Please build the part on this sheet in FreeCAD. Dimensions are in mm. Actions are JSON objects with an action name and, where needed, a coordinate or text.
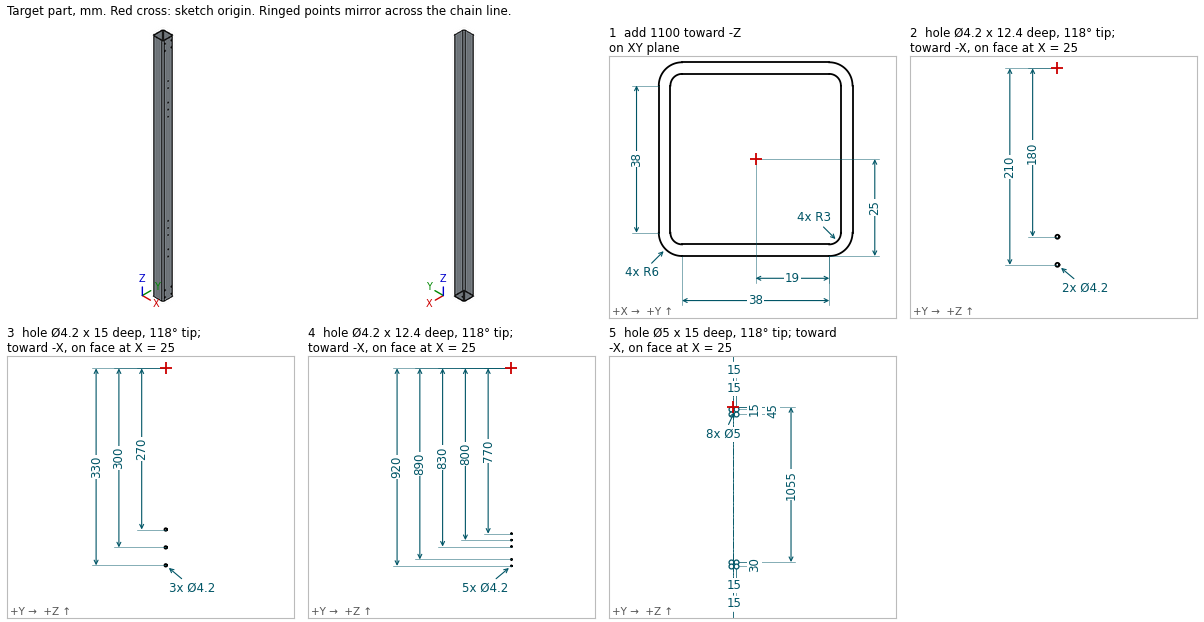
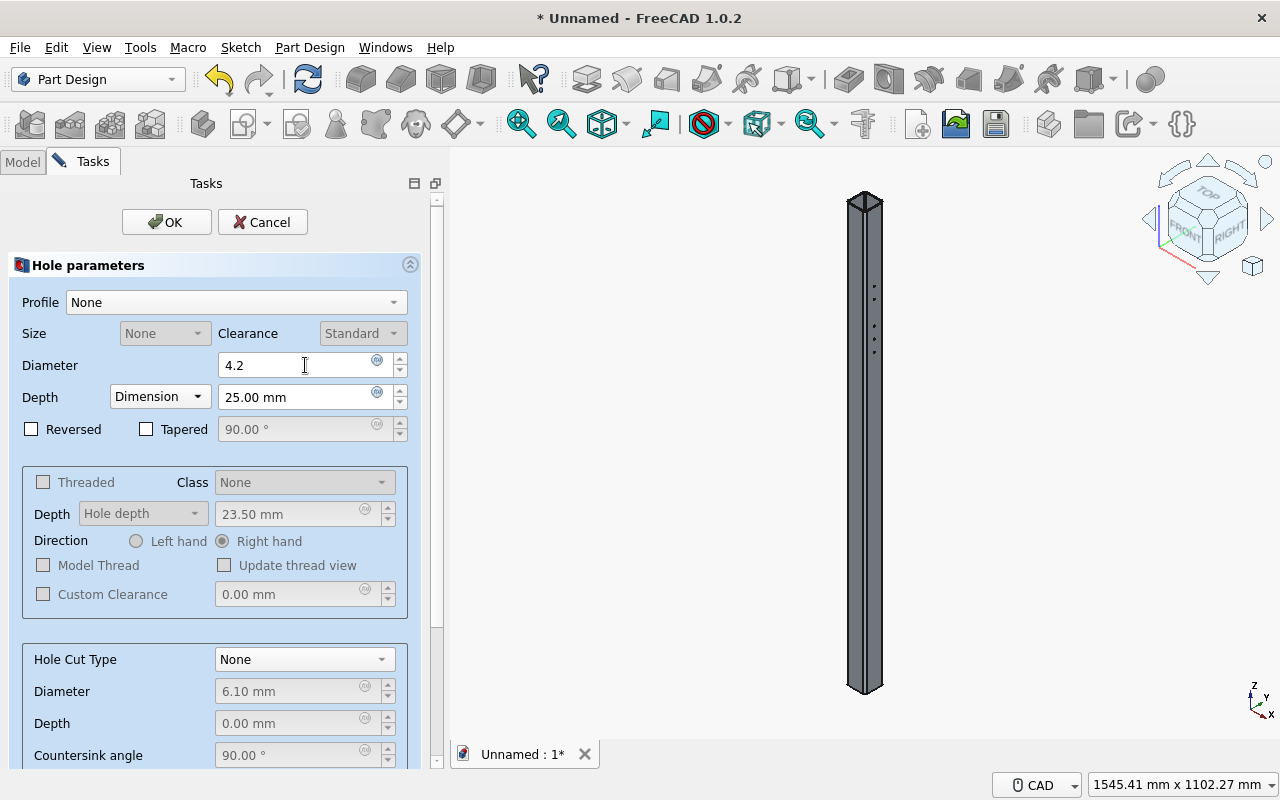
{"action": "triple_click", "coordinate": [305, 397]}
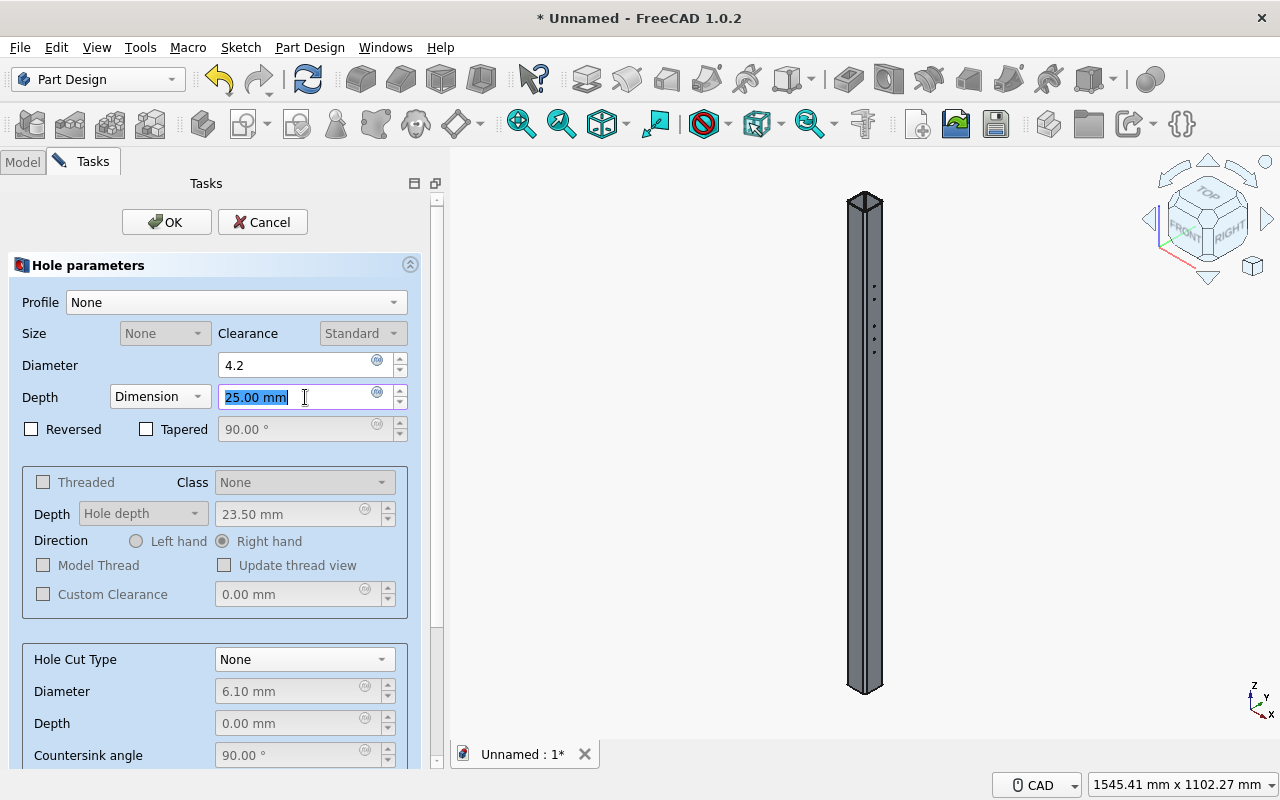
{"action": "type", "text": "15"}
{"action": "key", "text": "Tab"}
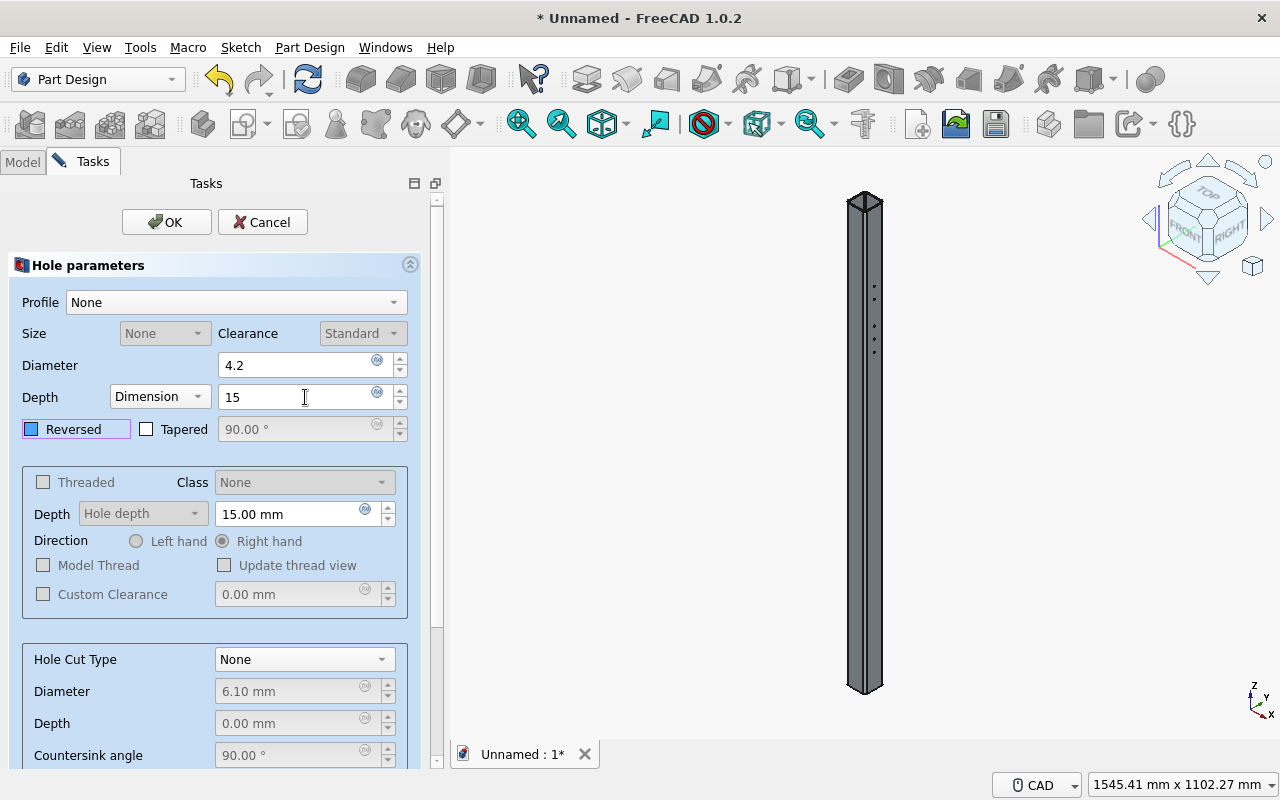
{"action": "left_click", "coordinate": [167, 222]}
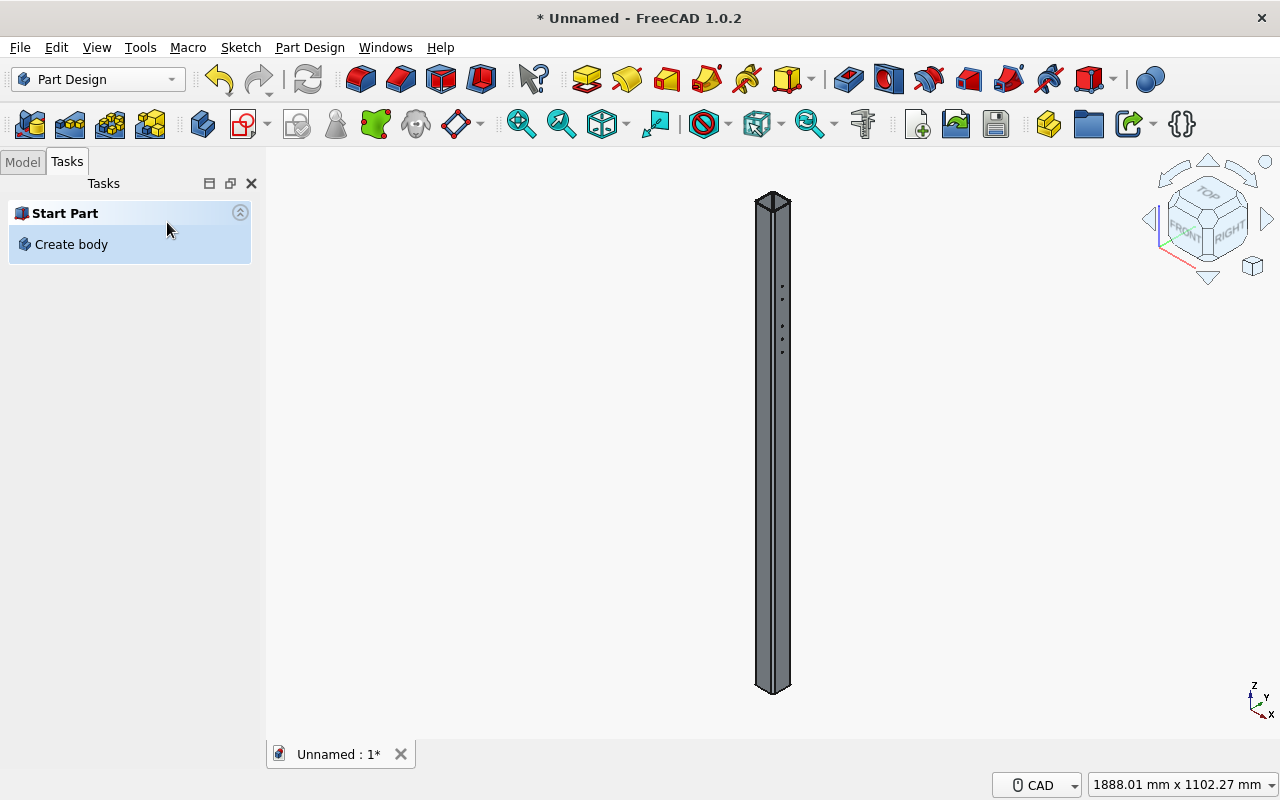
{"action": "left_click", "coordinate": [785, 240]}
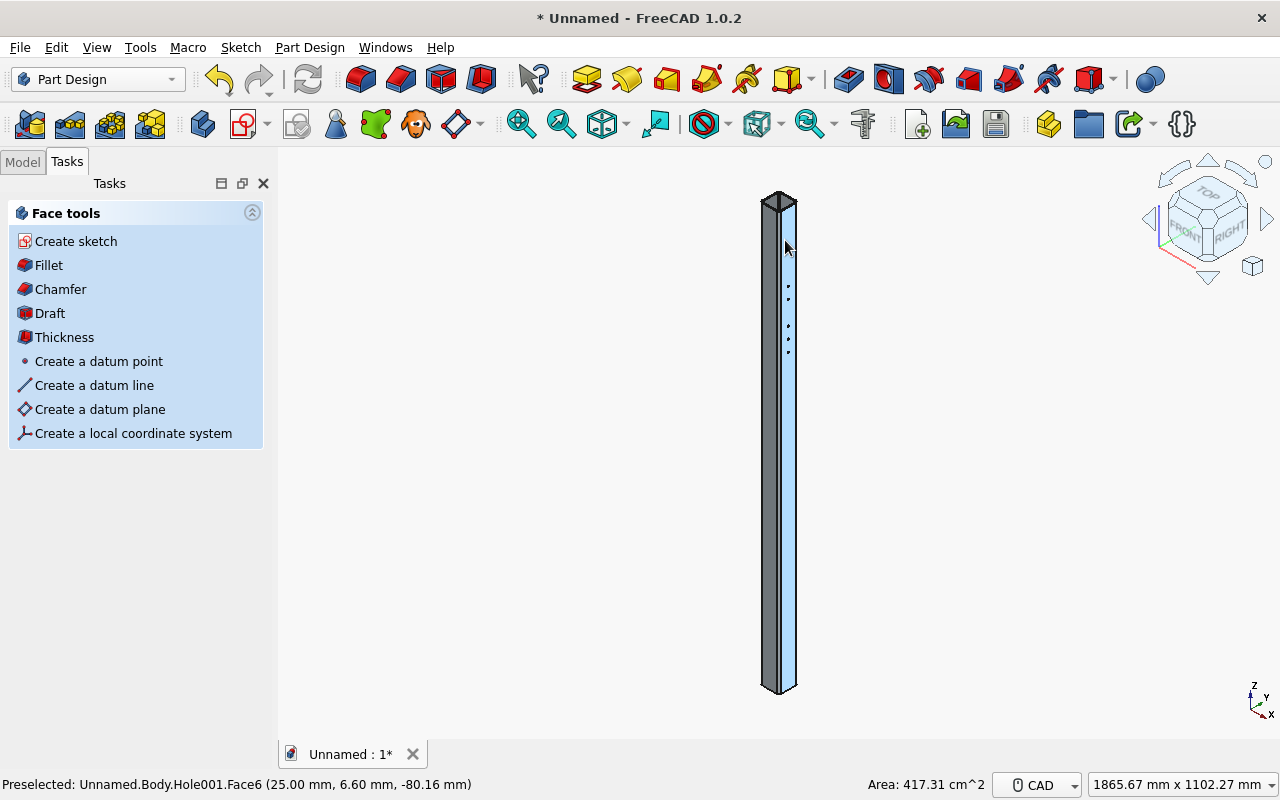
{"action": "left_click", "coordinate": [244, 124]}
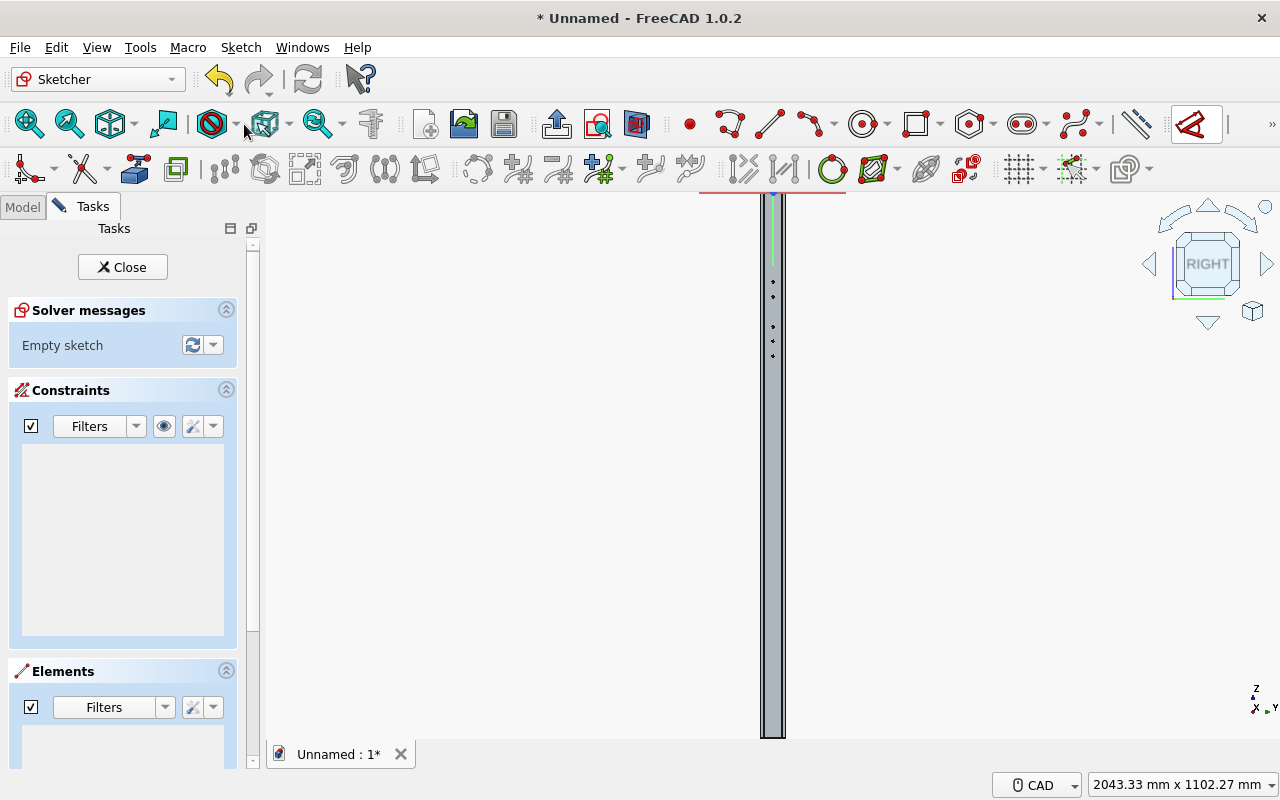
{"action": "scroll", "coordinate": [790, 649], "scroll_direction": "up", "scroll_amount": 8}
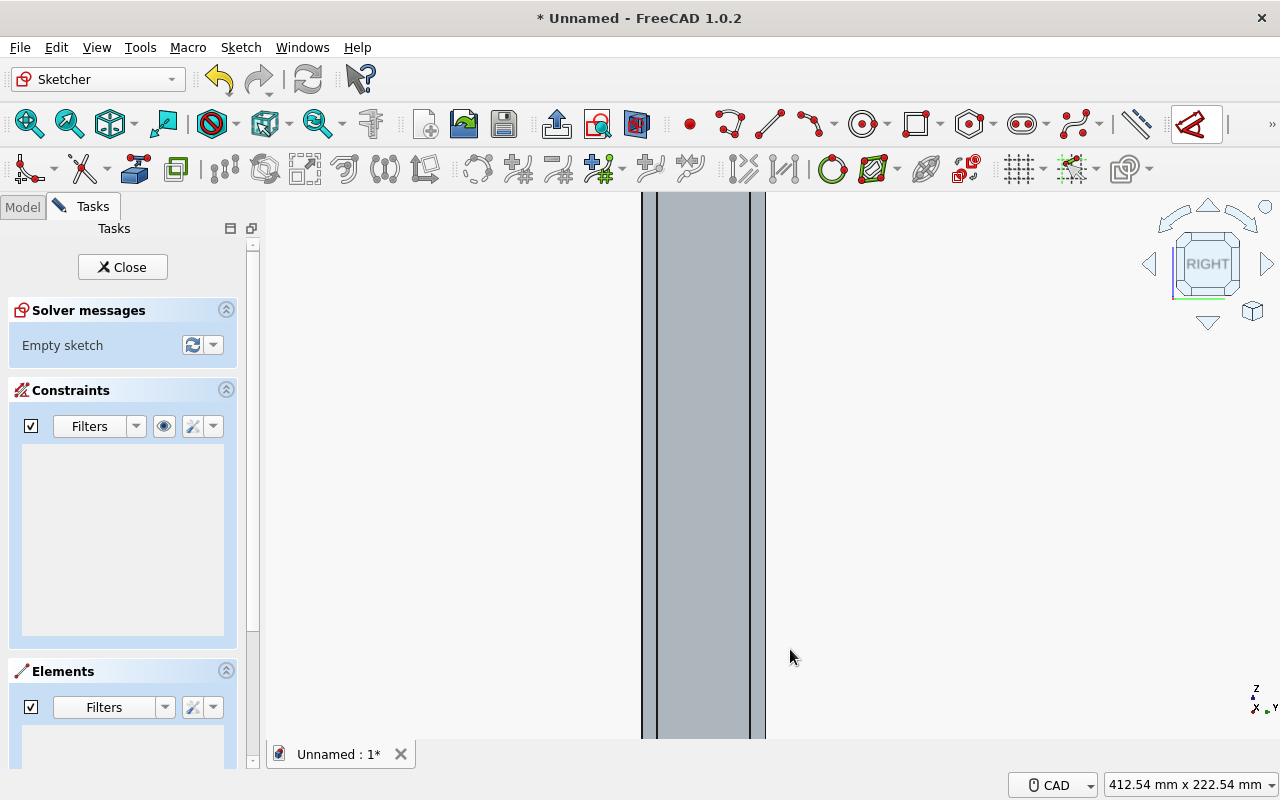
{"action": "left_click", "coordinate": [864, 124]}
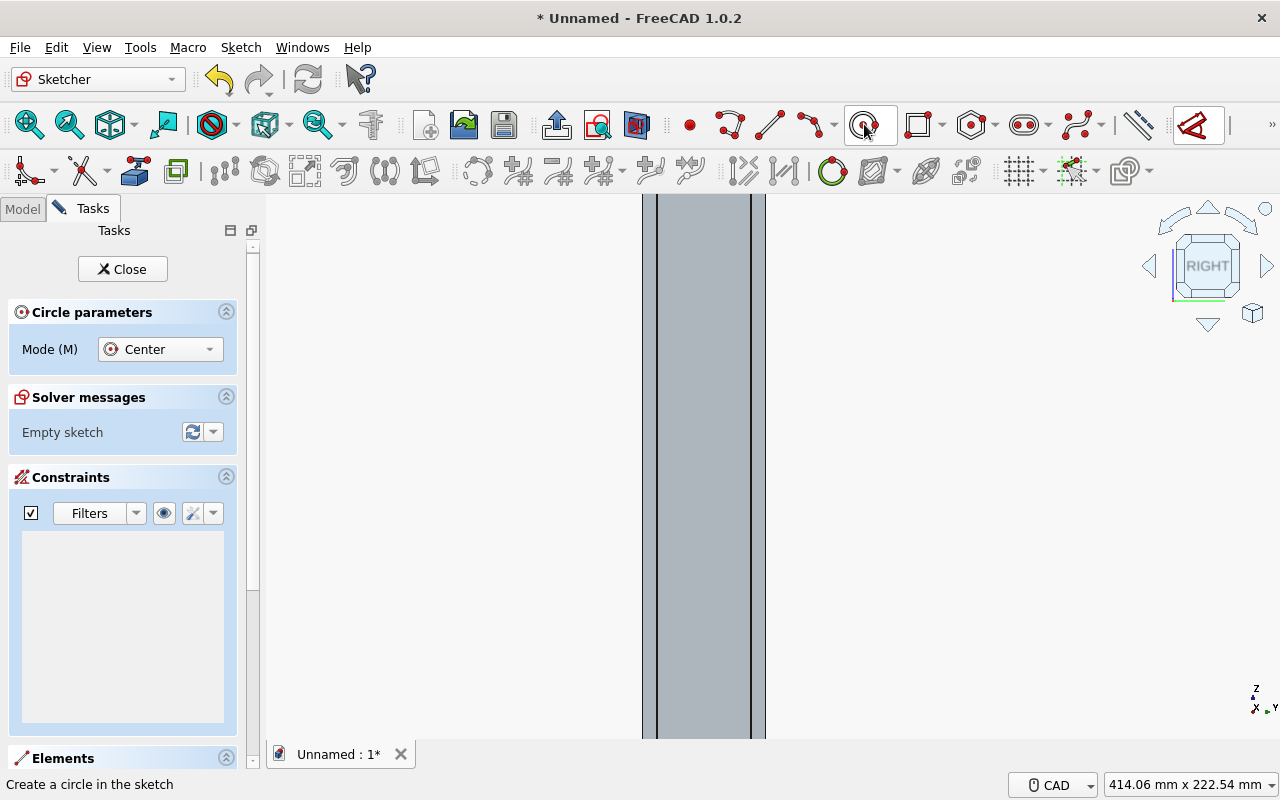
{"action": "scroll", "coordinate": [704, 647], "scroll_direction": "up", "scroll_amount": 8}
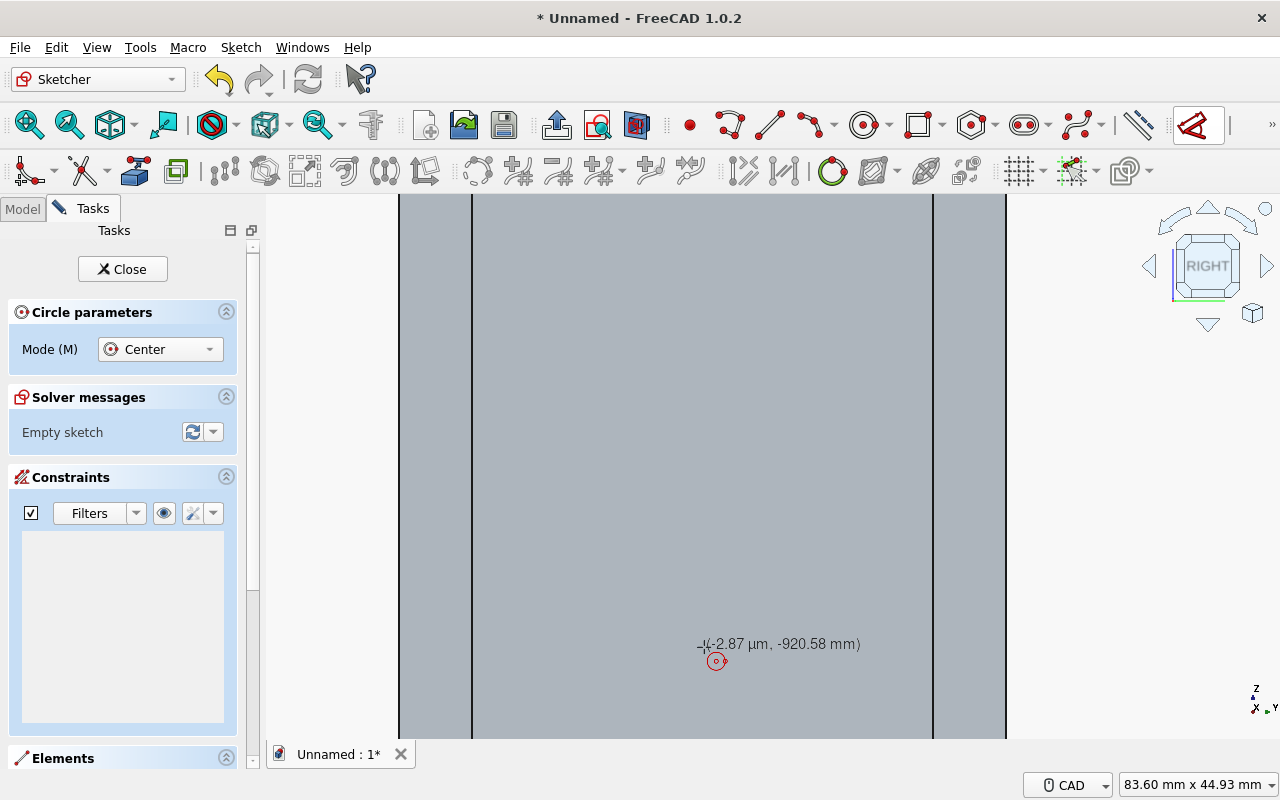
{"action": "scroll", "coordinate": [705, 652], "scroll_direction": "down", "scroll_amount": 8}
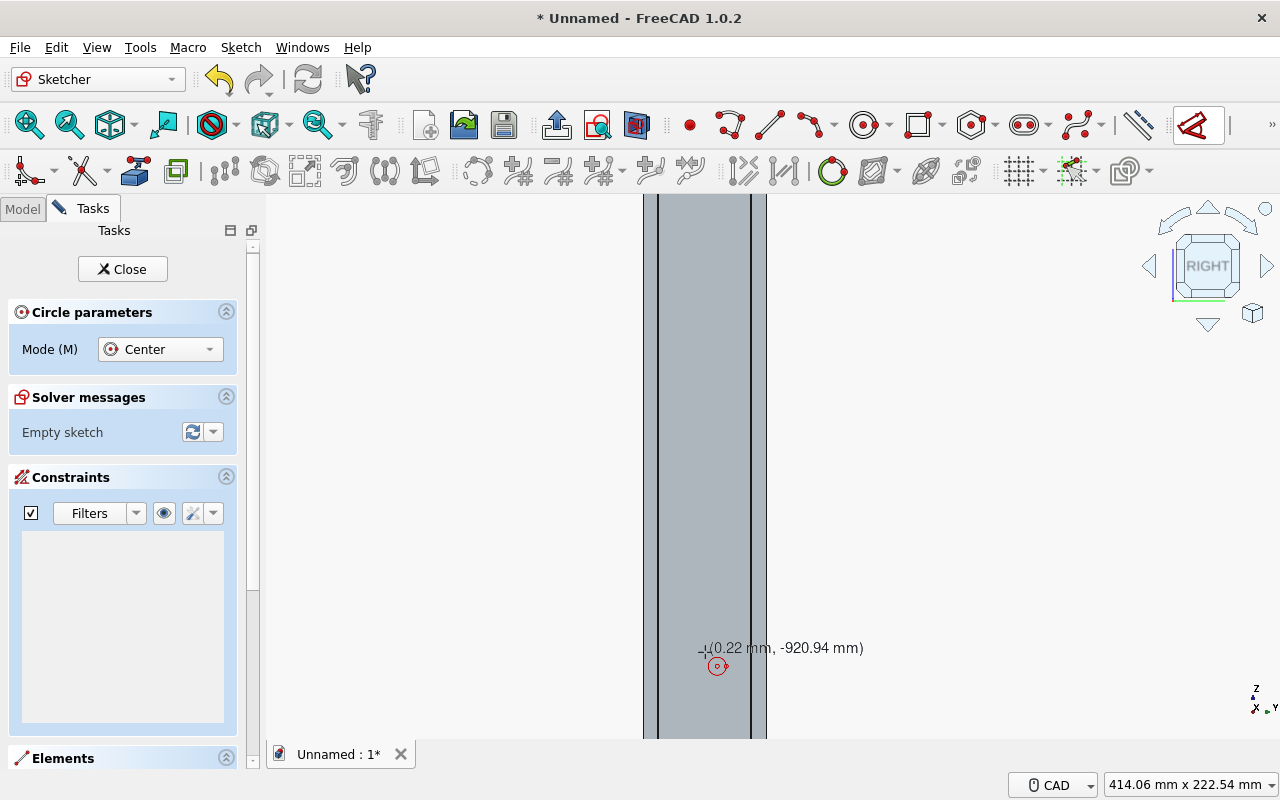
{"action": "left_click", "coordinate": [705, 651]}